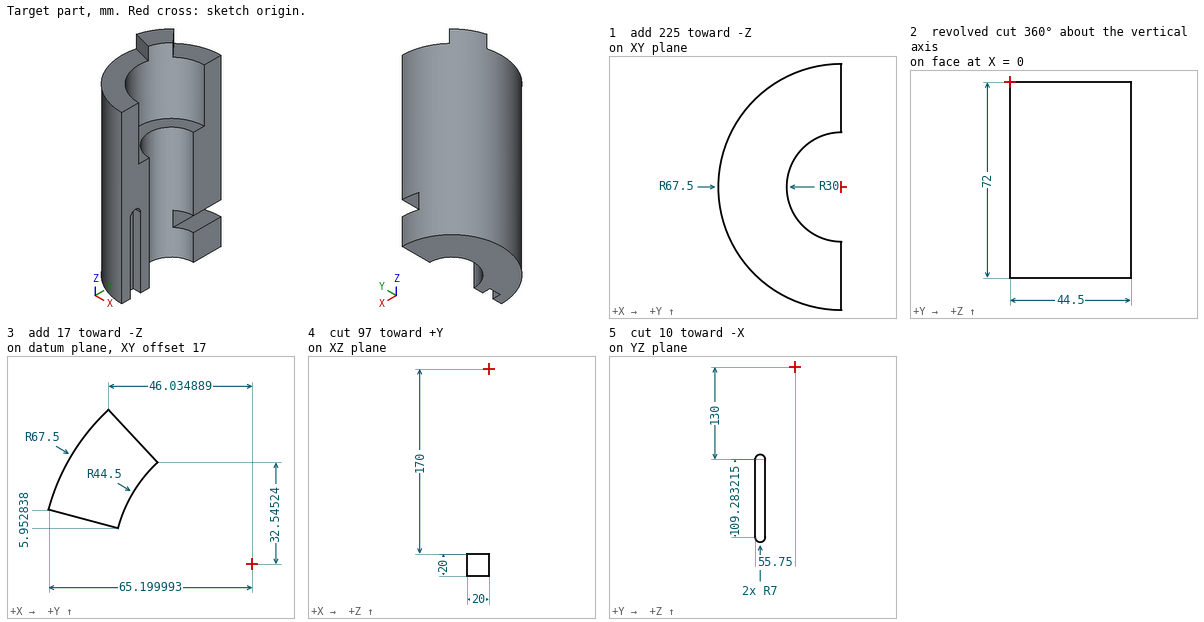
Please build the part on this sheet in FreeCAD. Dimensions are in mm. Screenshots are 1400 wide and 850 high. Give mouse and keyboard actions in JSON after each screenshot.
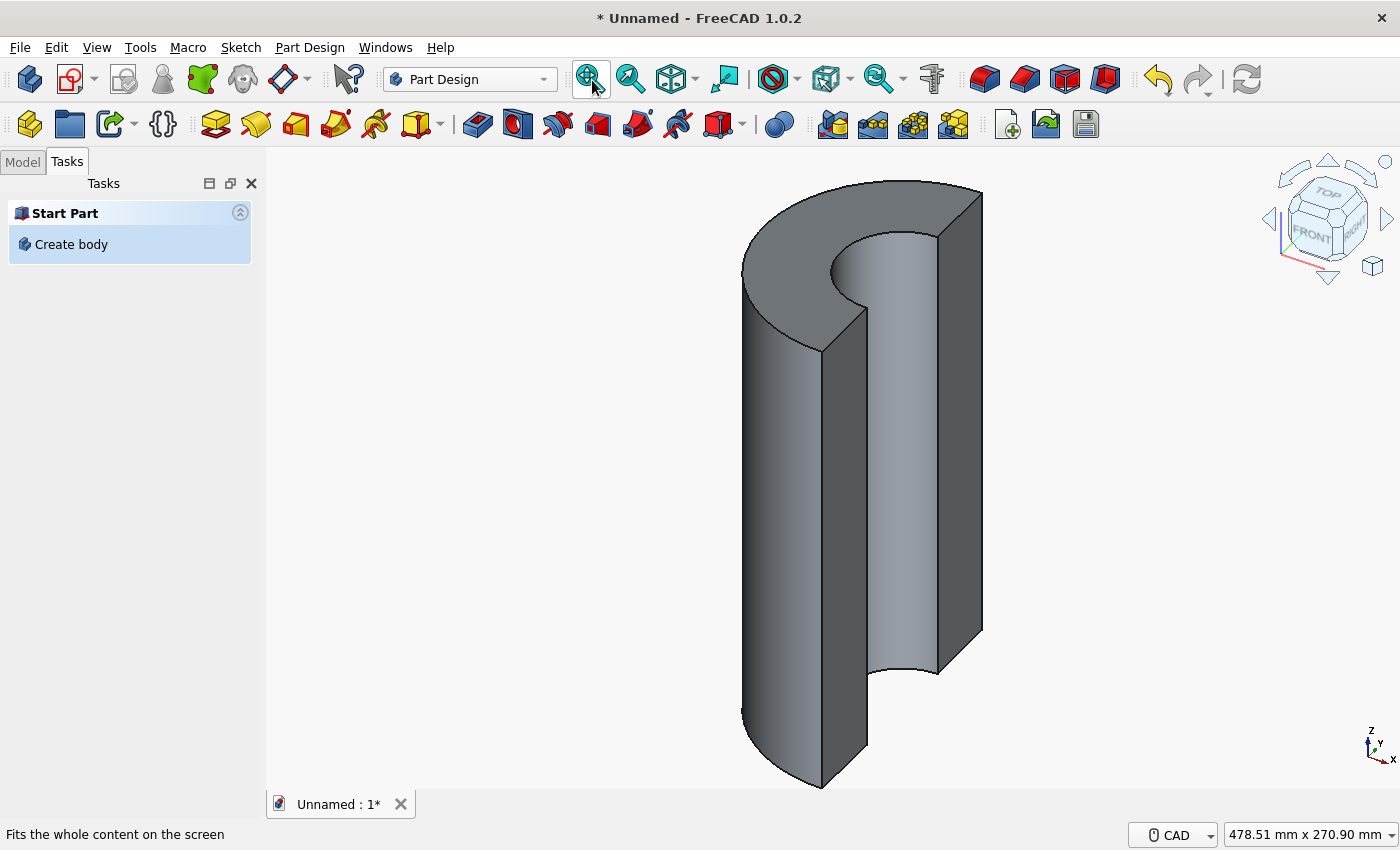
{"action": "left_click", "coordinate": [844, 422]}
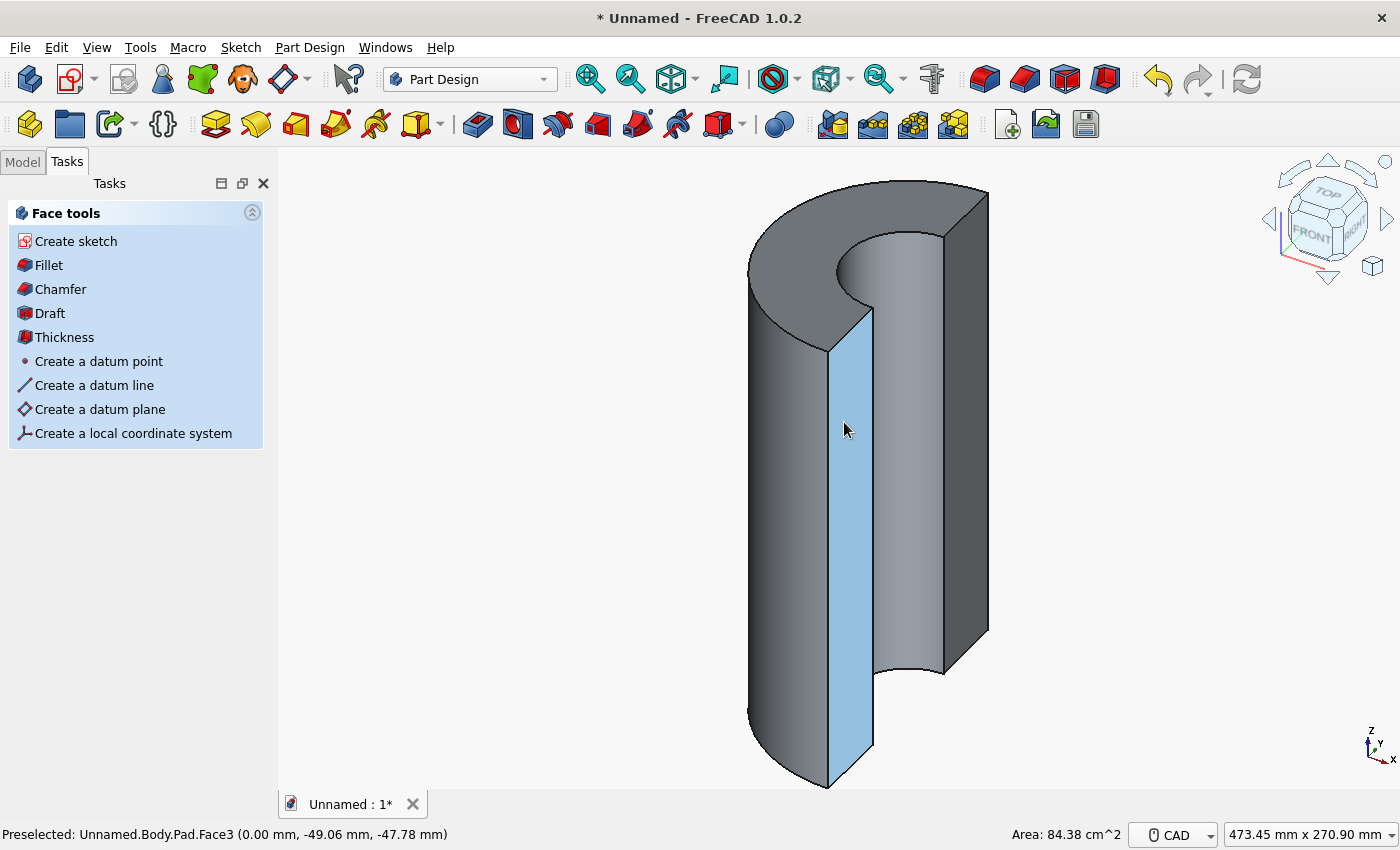
{"action": "left_click", "coordinate": [70, 80]}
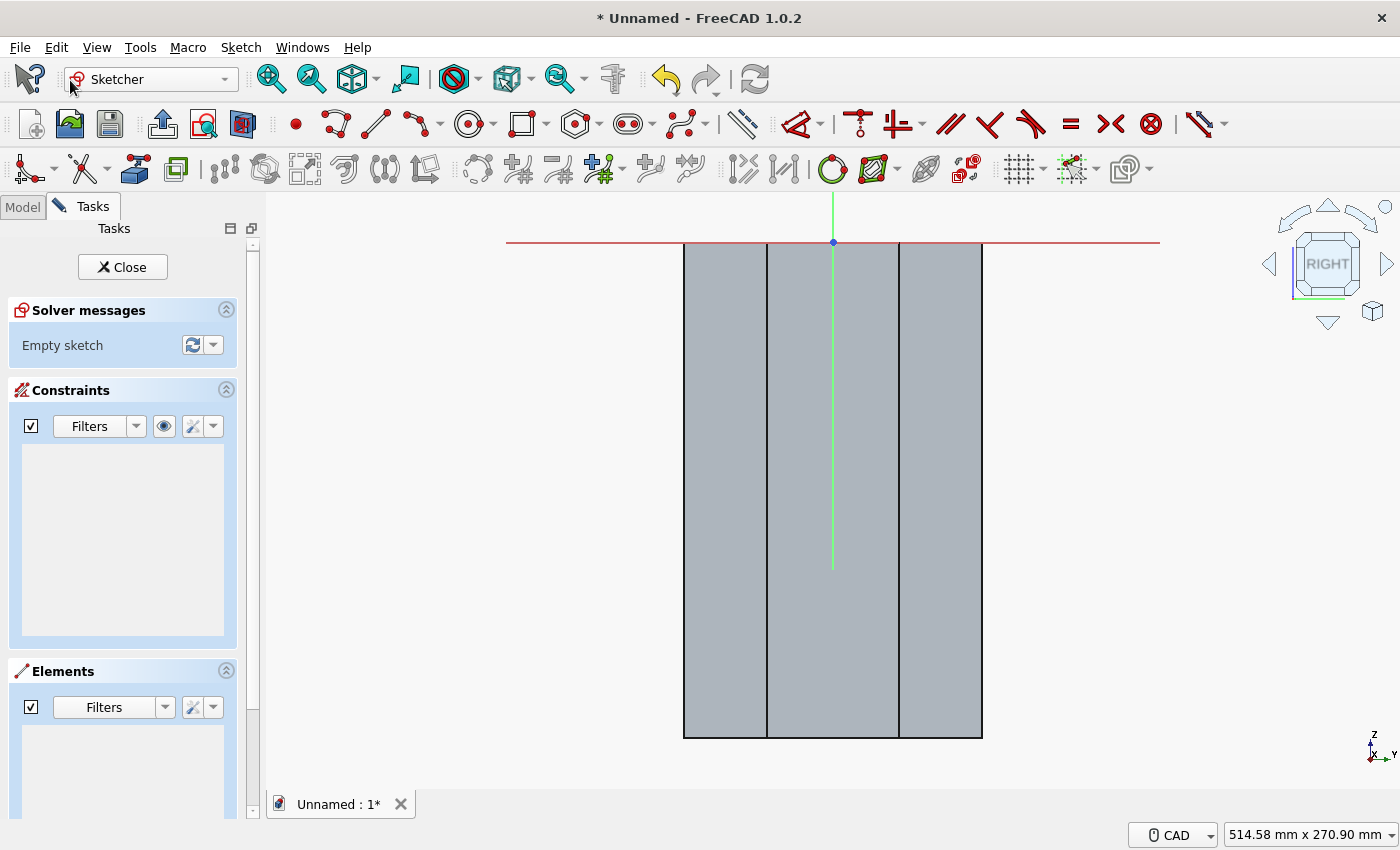
{"action": "scroll", "coordinate": [978, 220], "scroll_direction": "up", "scroll_amount": 4}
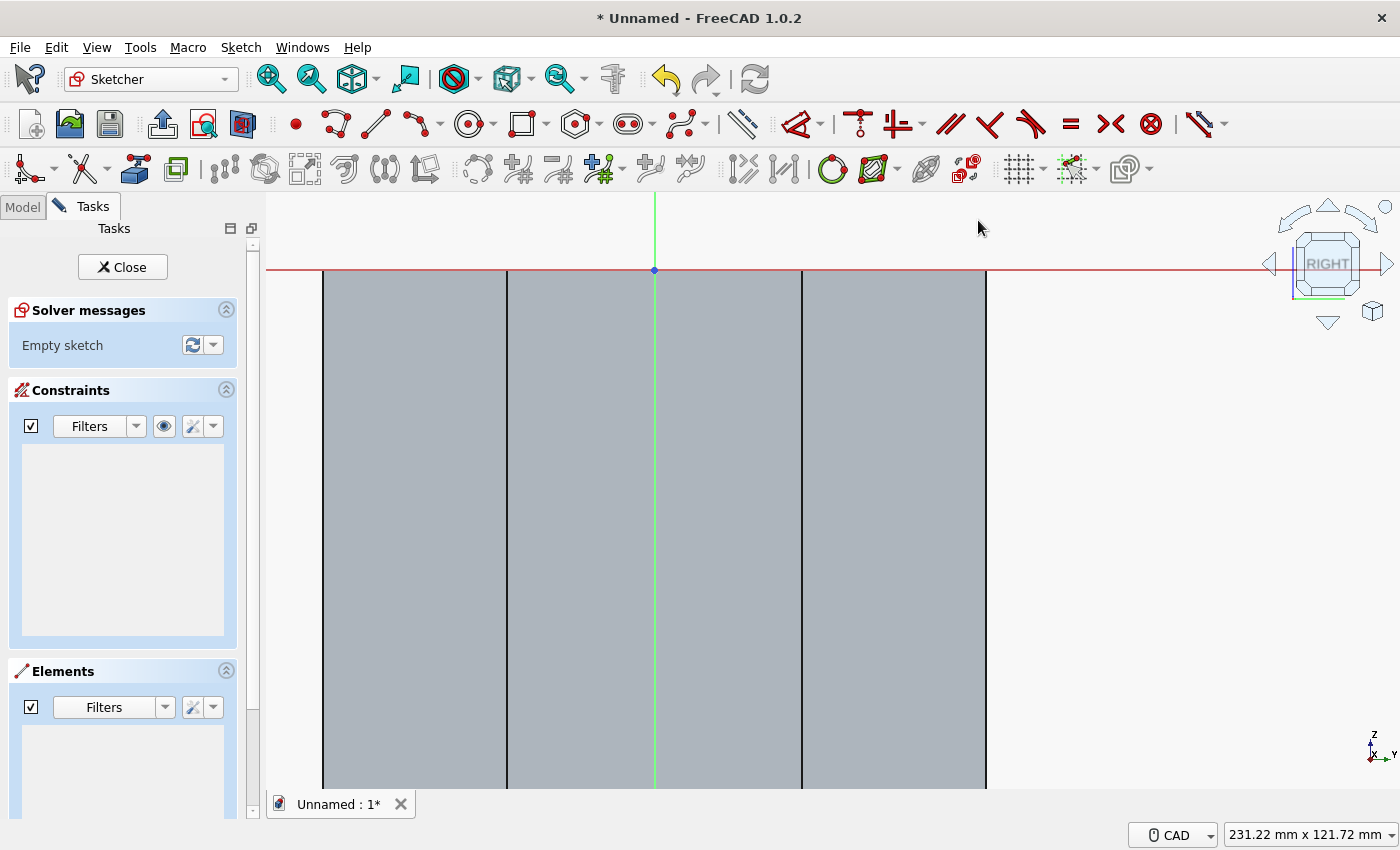
{"action": "key", "text": "g r"}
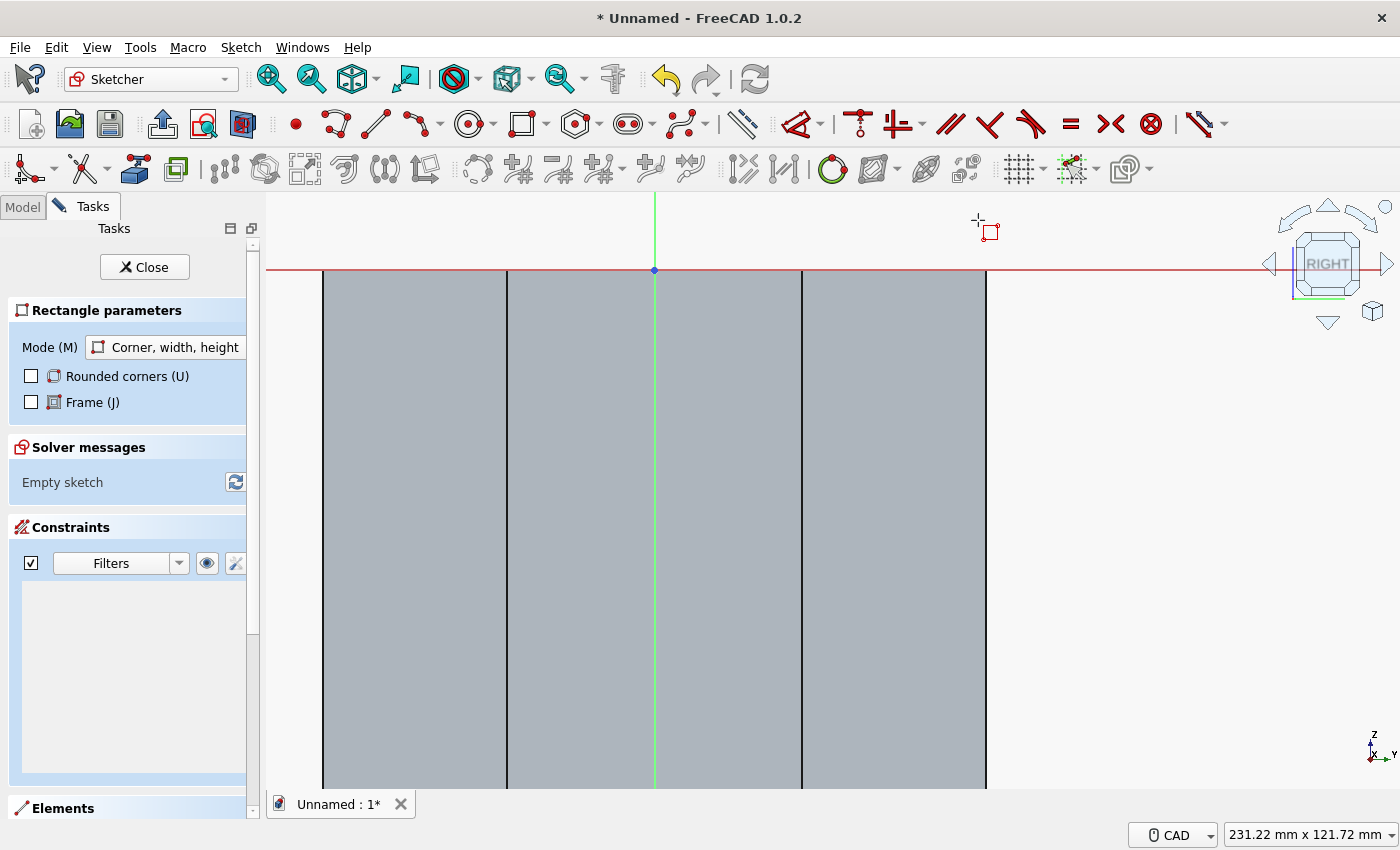
{"action": "left_click", "coordinate": [655, 270]}
{"action": "left_click", "coordinate": [873, 623]}
{"action": "key", "text": "Escape"}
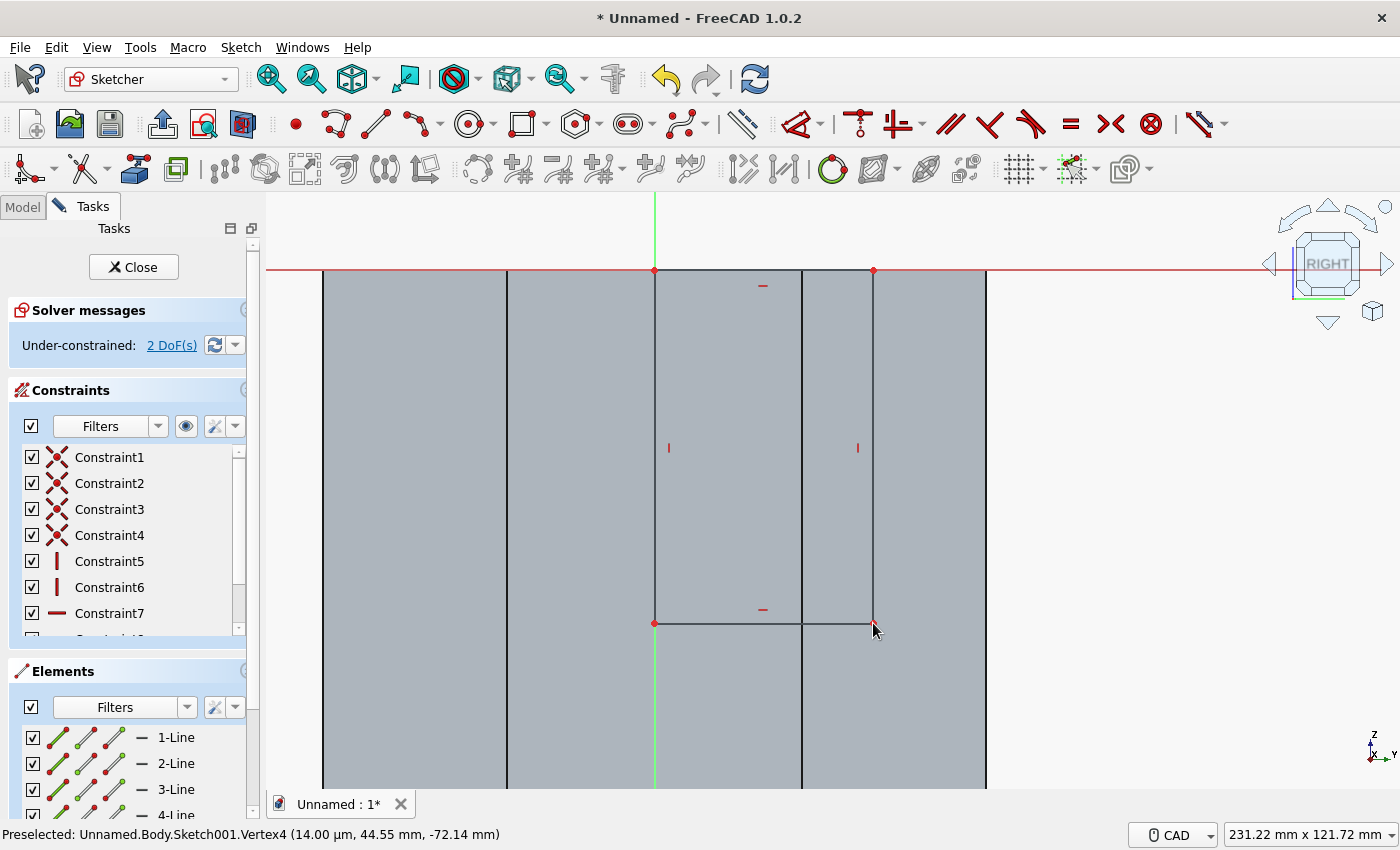
{"action": "left_click", "coordinate": [655, 376]}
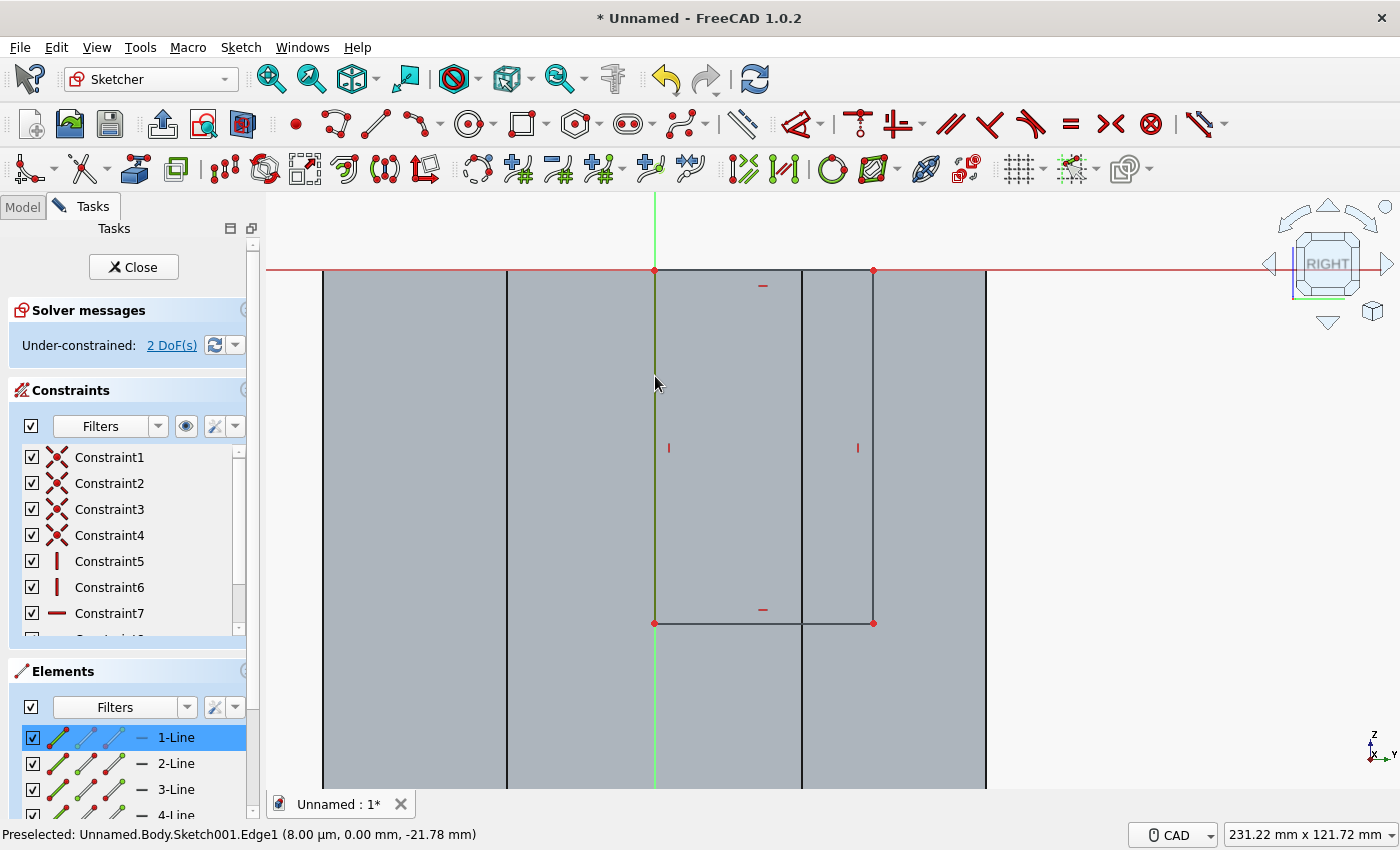
{"action": "key", "text": "i"}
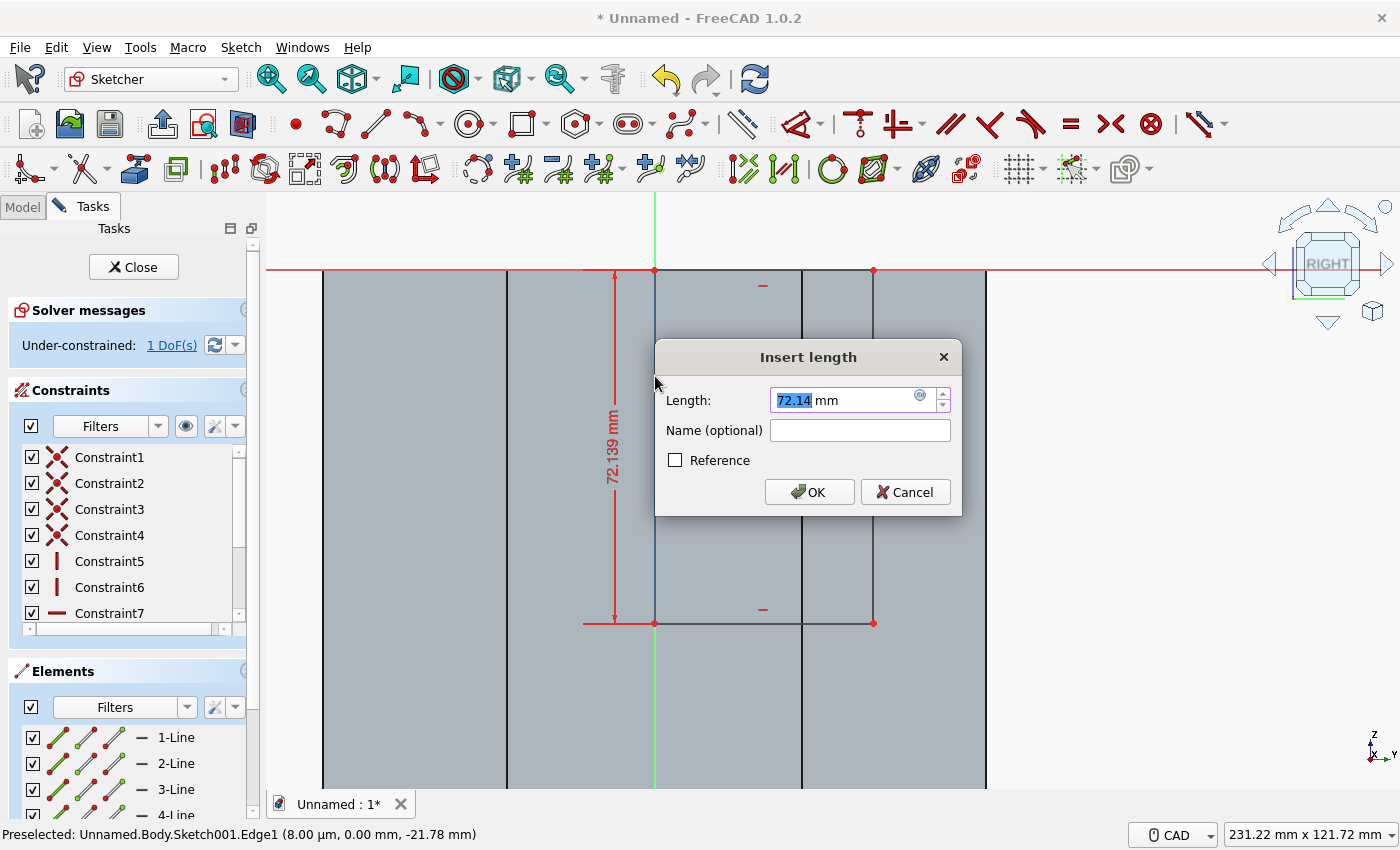
{"action": "type", "text": "72"}
{"action": "key", "text": "Return"}